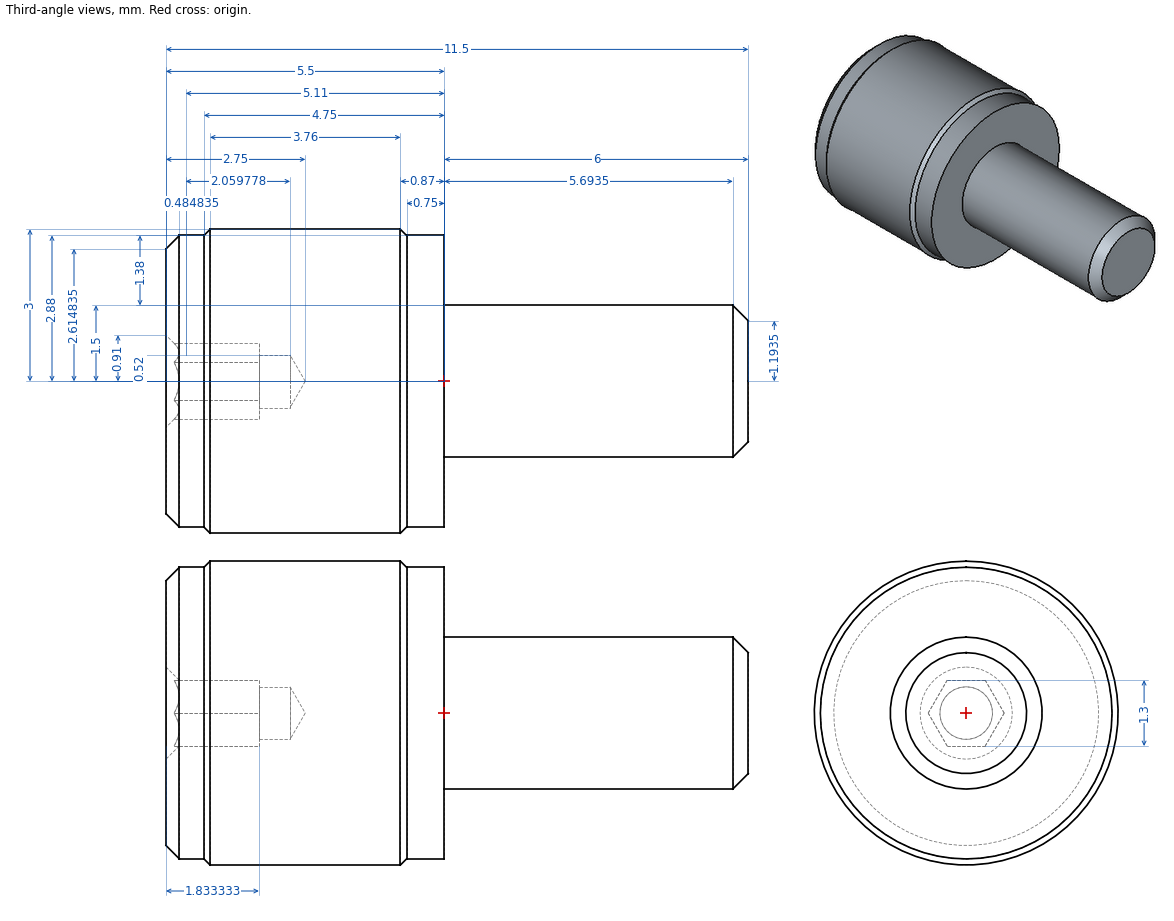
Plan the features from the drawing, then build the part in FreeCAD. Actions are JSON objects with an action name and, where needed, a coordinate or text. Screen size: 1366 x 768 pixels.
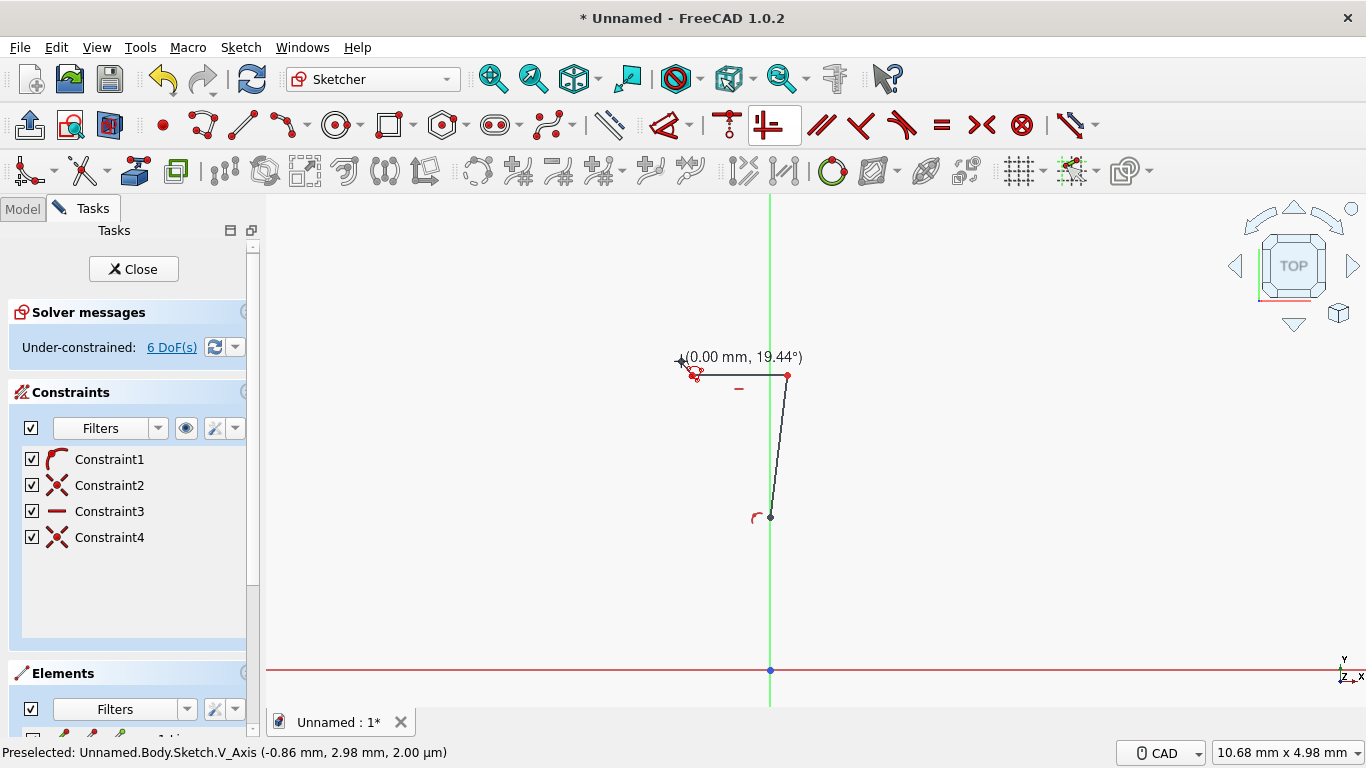
{"action": "scroll", "coordinate": [688, 371], "scroll_direction": "down", "scroll_amount": 3}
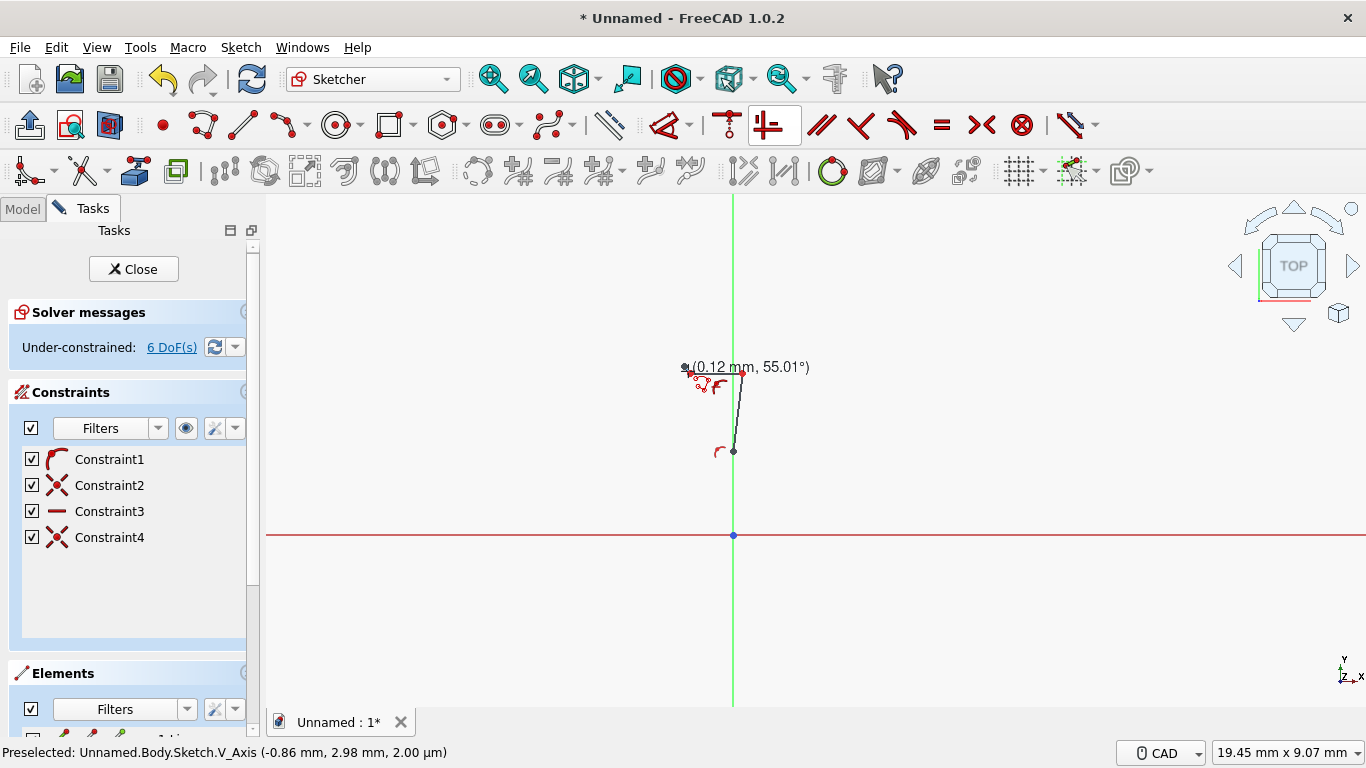
{"action": "left_click", "coordinate": [472, 366]}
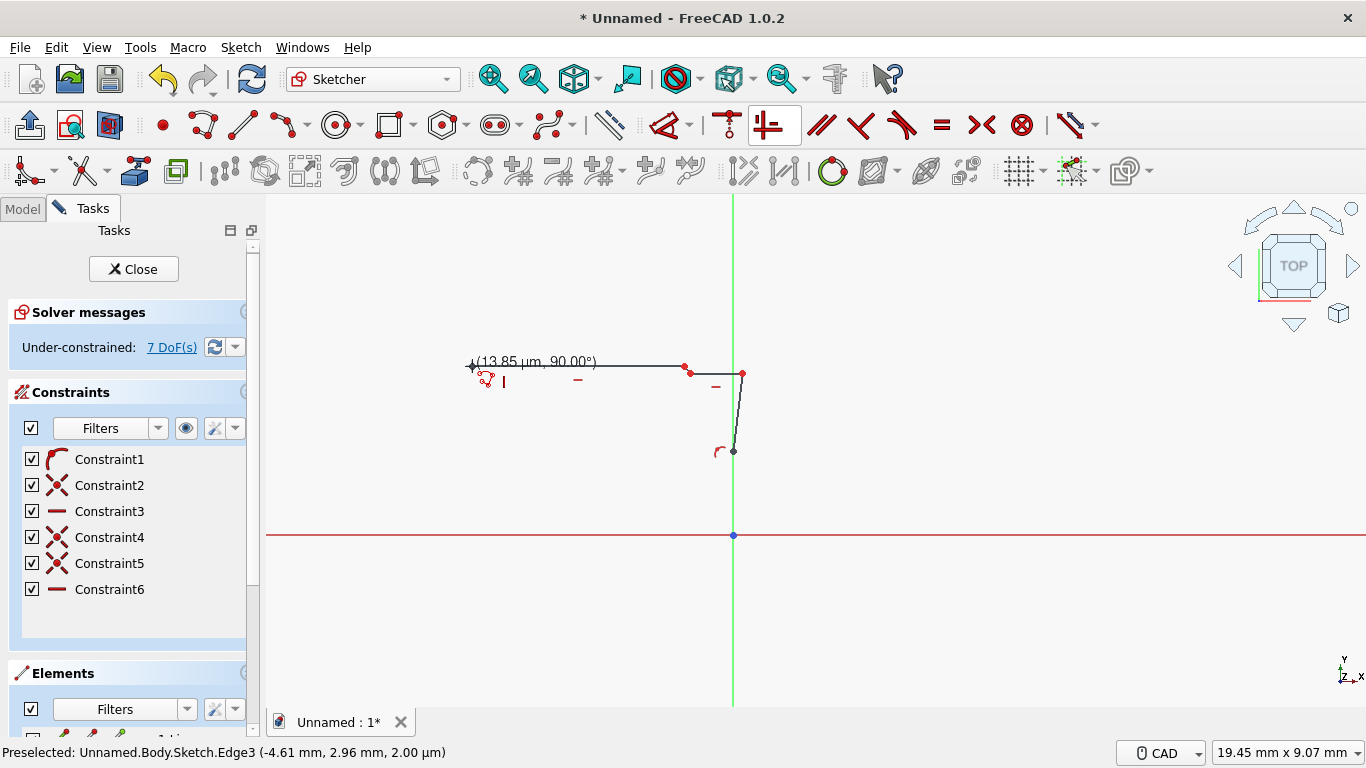
{"action": "scroll", "coordinate": [465, 373], "scroll_direction": "up", "scroll_amount": 3}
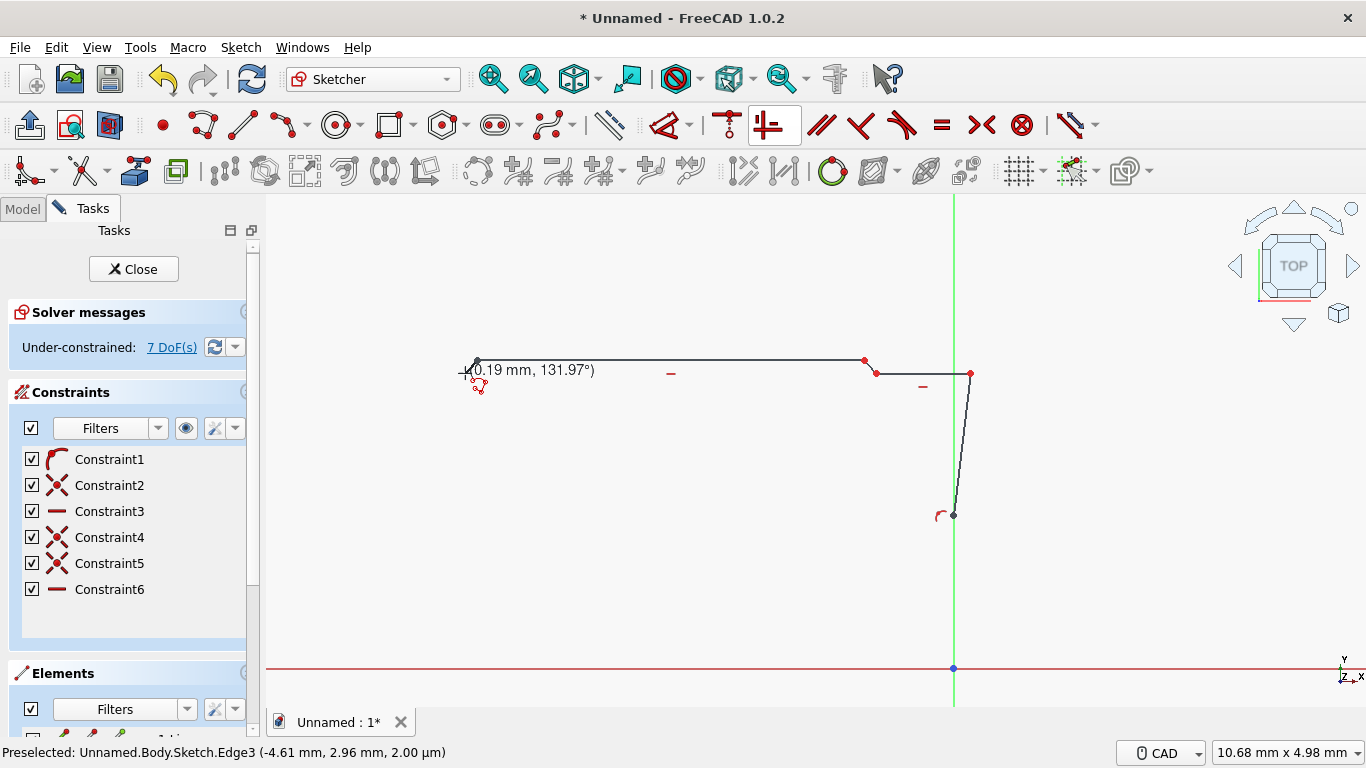
{"action": "left_click", "coordinate": [465, 372]}
{"action": "left_click", "coordinate": [415, 372]}
{"action": "left_click", "coordinate": [387, 399]}
{"action": "left_click", "coordinate": [387, 669]}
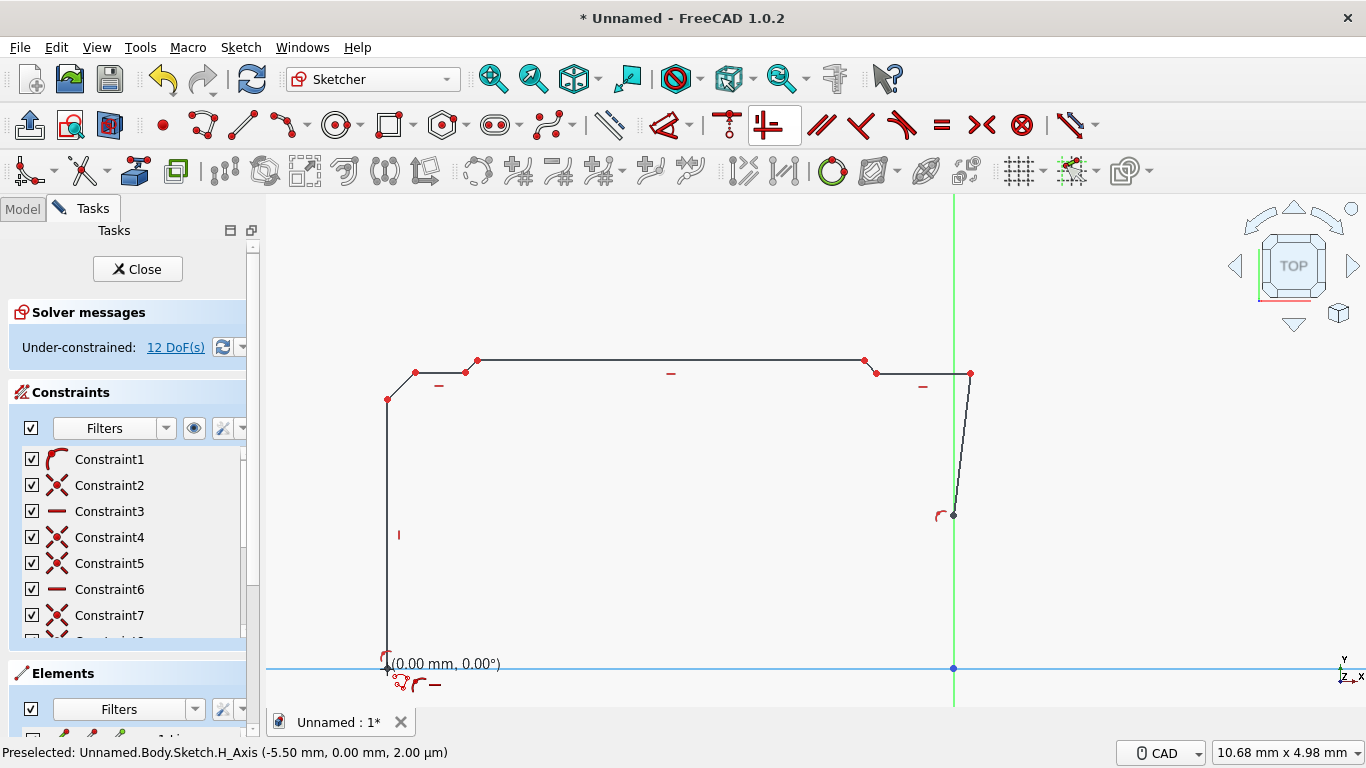
{"action": "scroll", "coordinate": [465, 373], "scroll_direction": "down", "scroll_amount": 3}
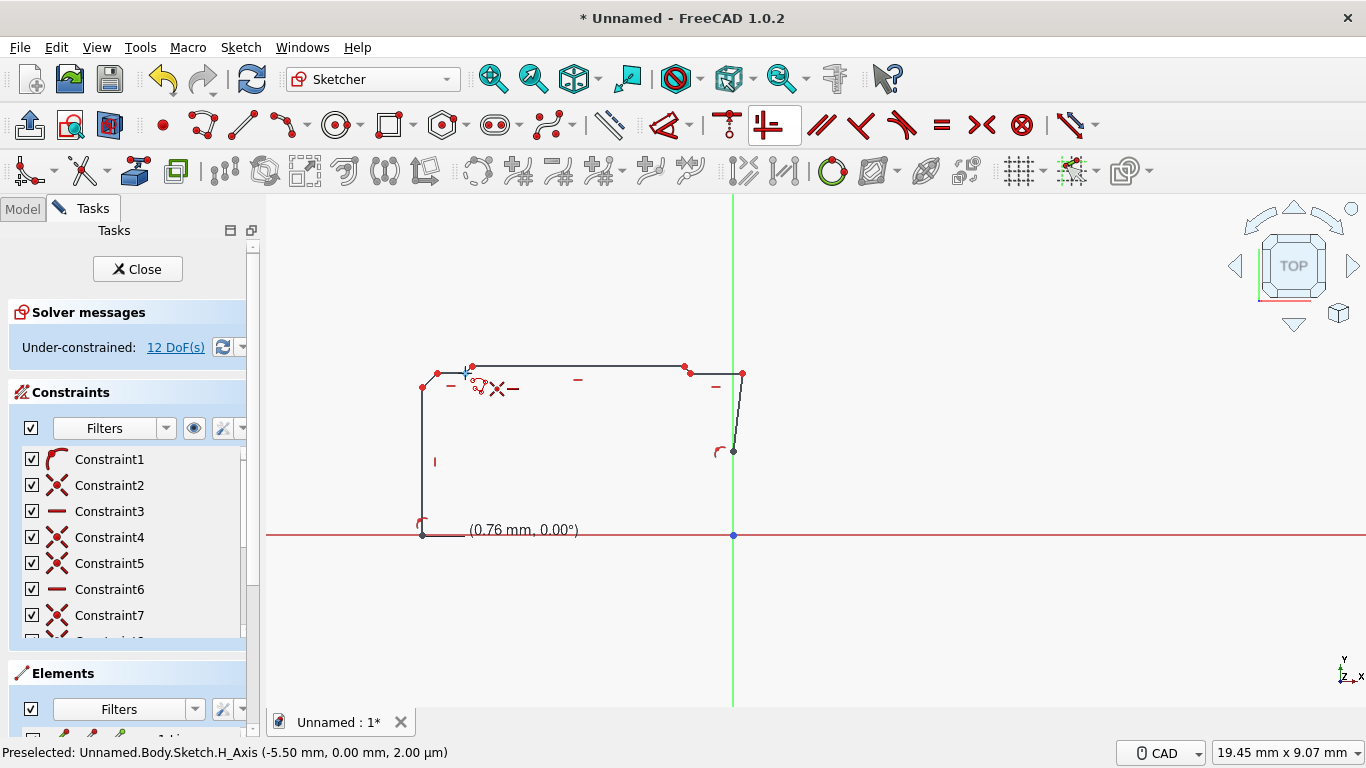
{"action": "left_click", "coordinate": [1073, 526]}
{"action": "left_click", "coordinate": [1073, 468]}
{"action": "left_click", "coordinate": [1055, 451]}
{"action": "left_click", "coordinate": [733, 452]}
{"action": "key", "text": "Escape"}
{"action": "key", "text": "Escape"}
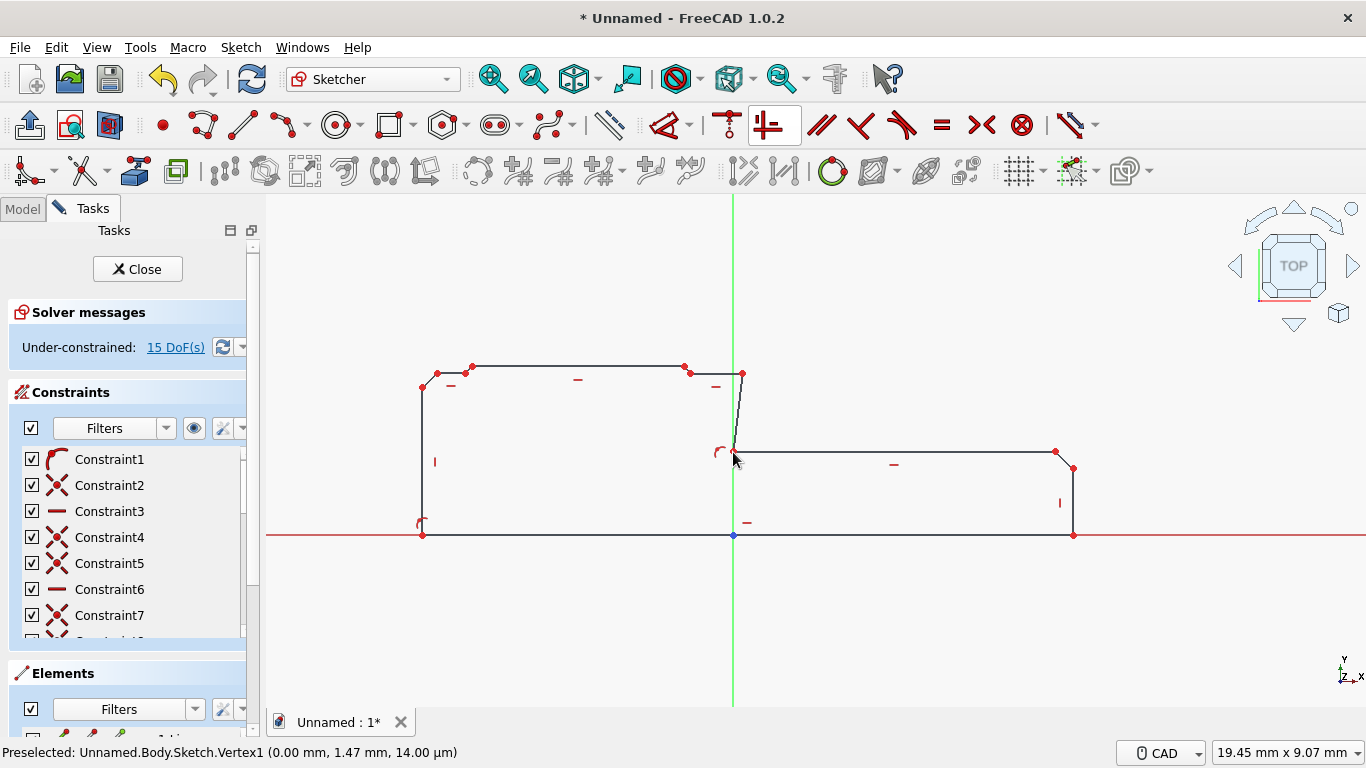
{"action": "left_click", "coordinate": [736, 428]}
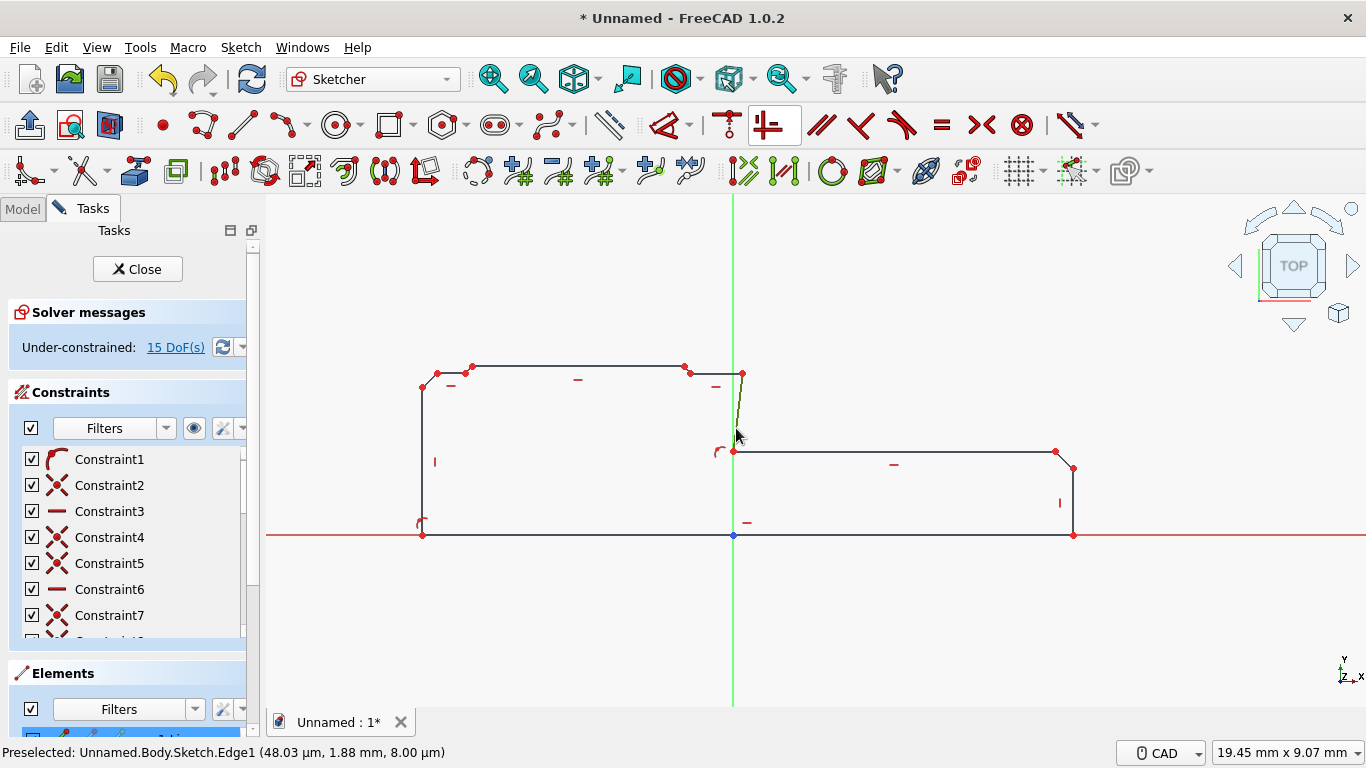
{"action": "key", "text": "v"}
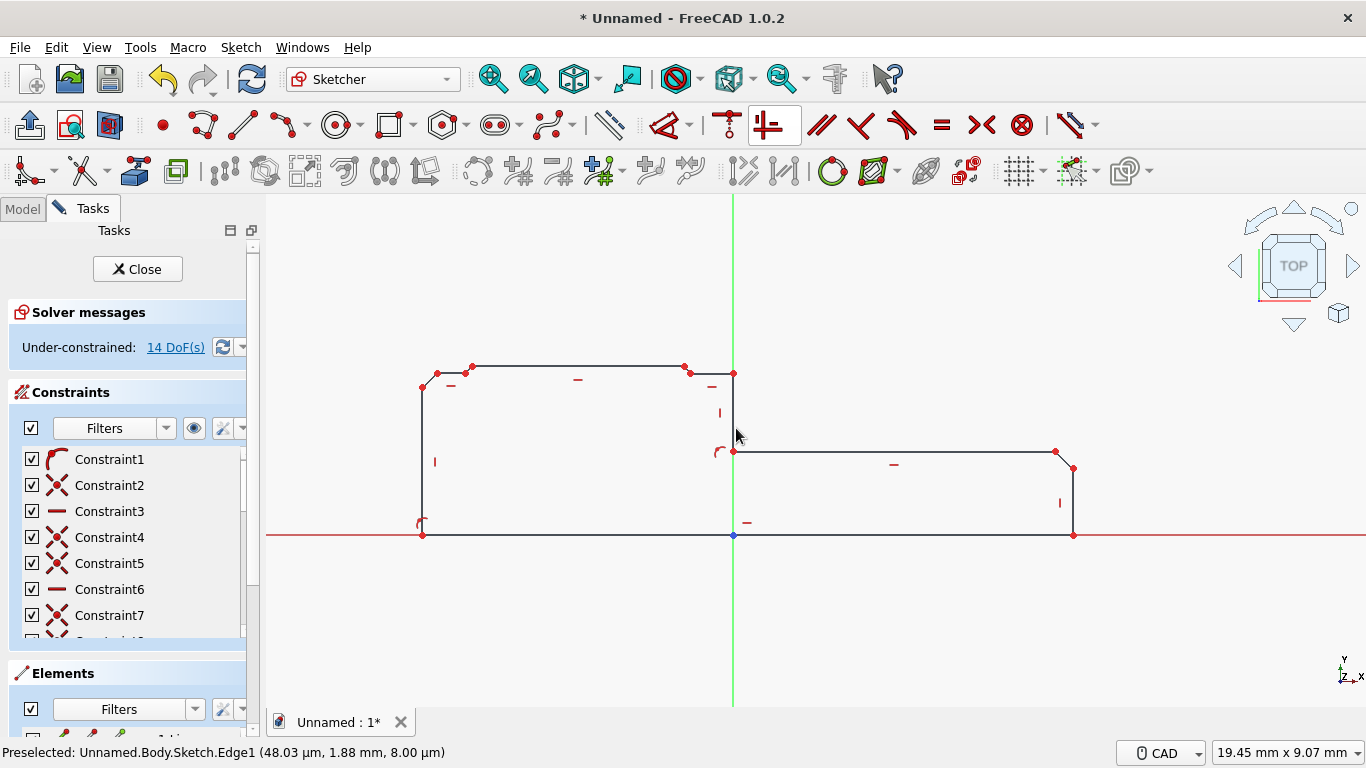
{"action": "left_click", "coordinate": [664, 126]}